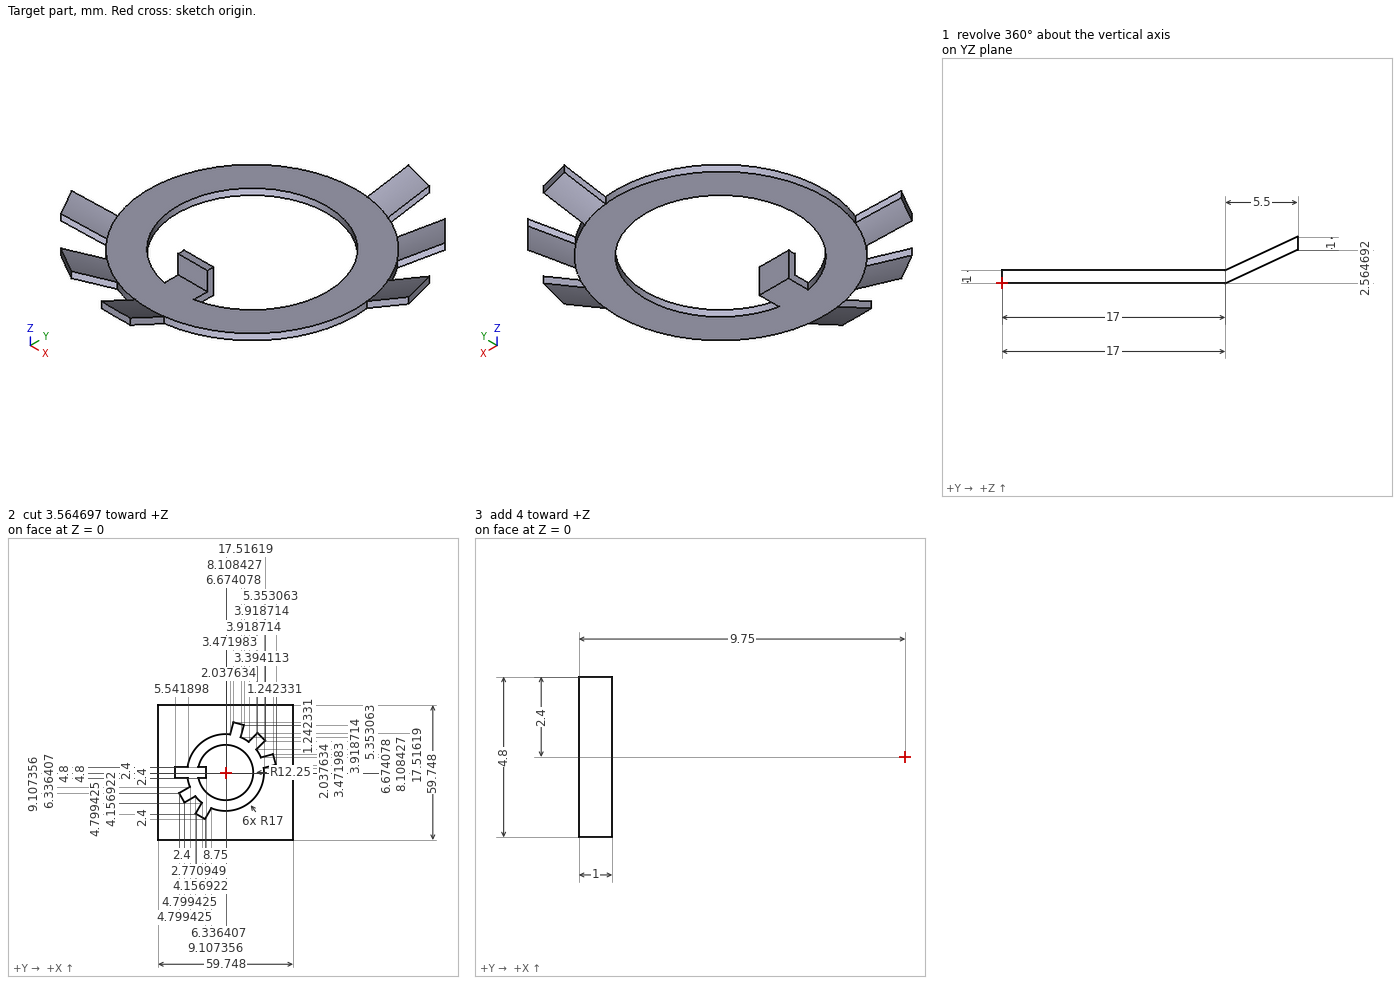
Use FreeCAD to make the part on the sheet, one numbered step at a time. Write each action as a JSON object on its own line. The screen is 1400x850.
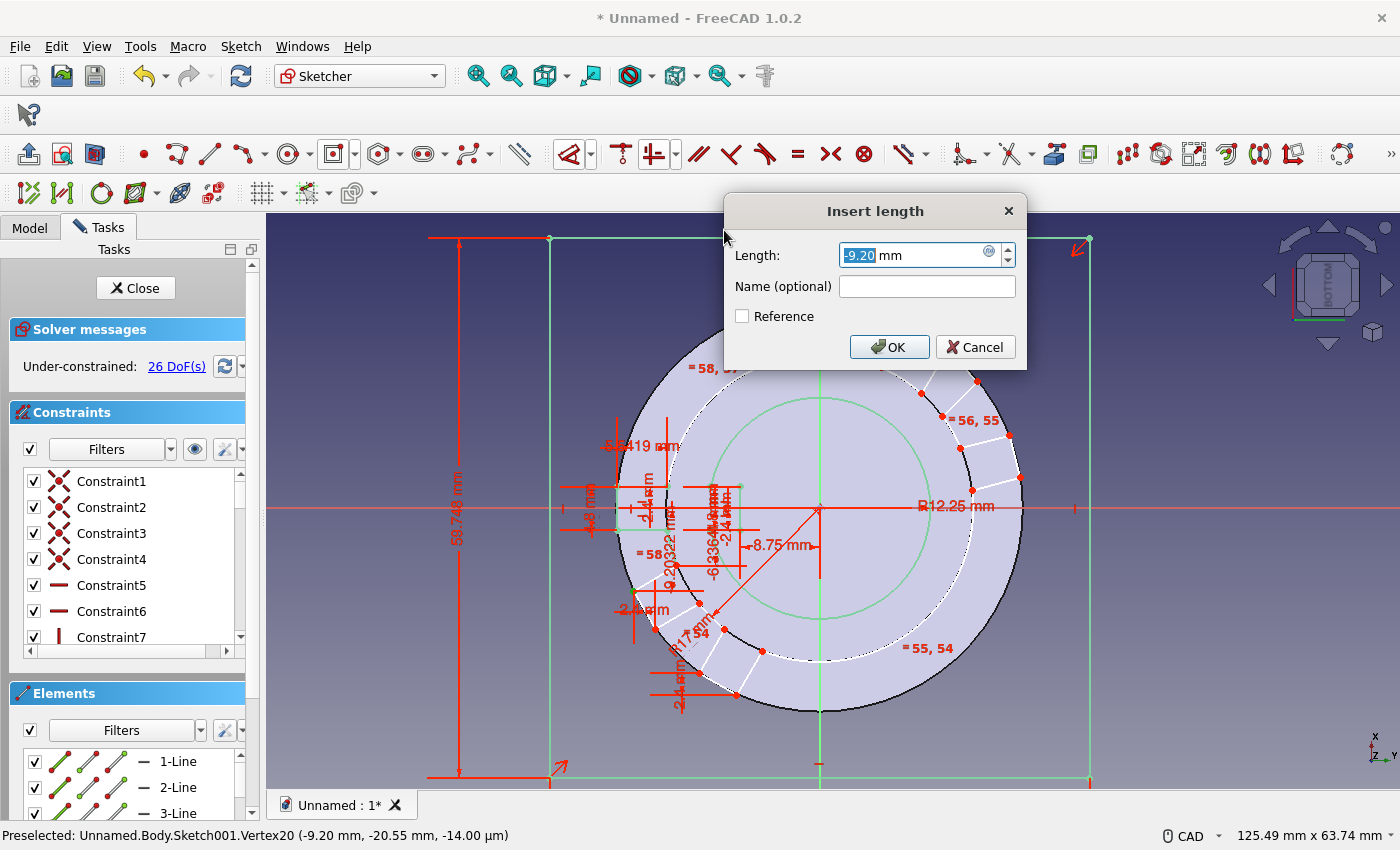
{"action": "type", "text": "-9.107356"}
{"action": "key", "text": "Return"}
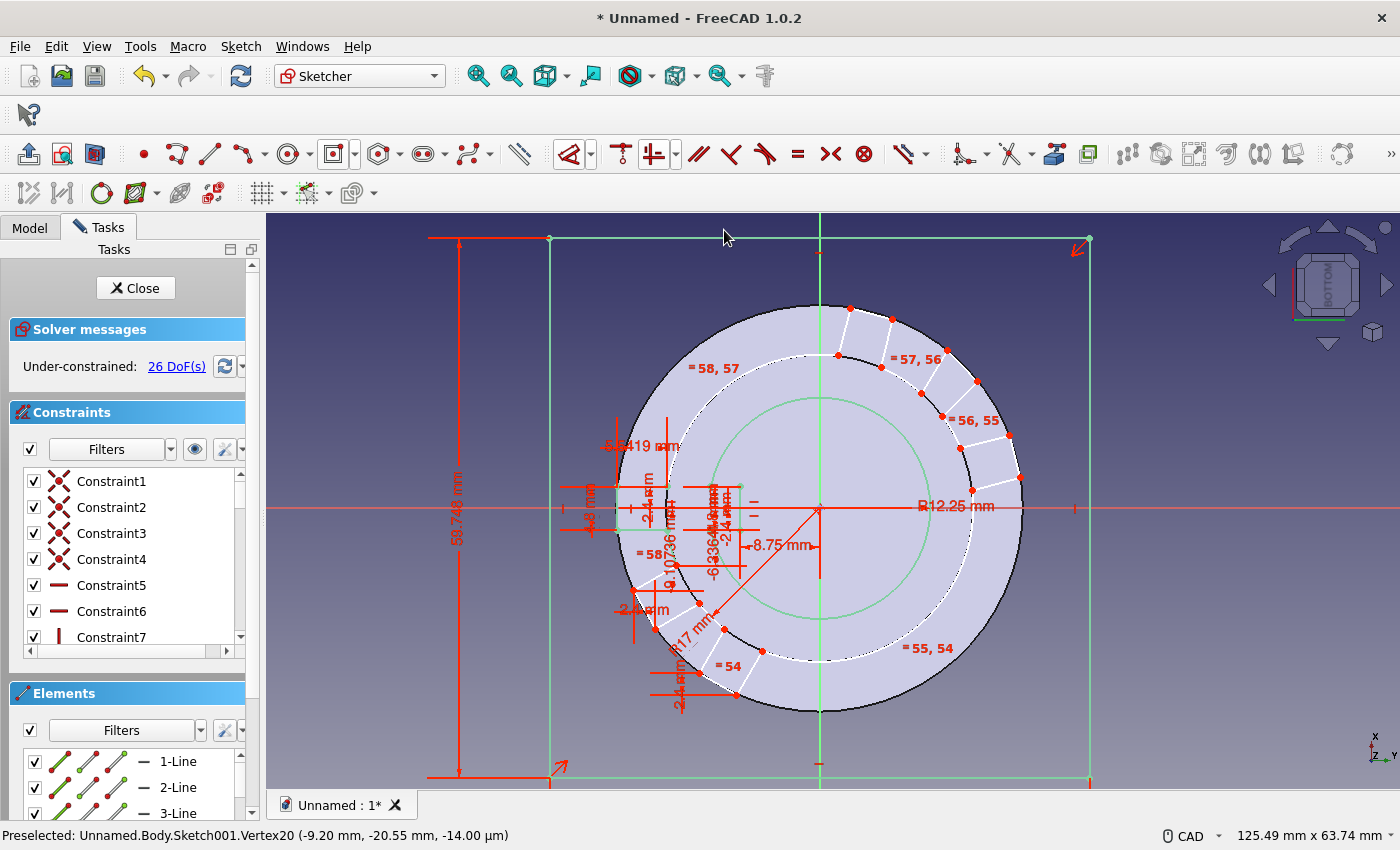
{"action": "left_click", "coordinate": [737, 695]}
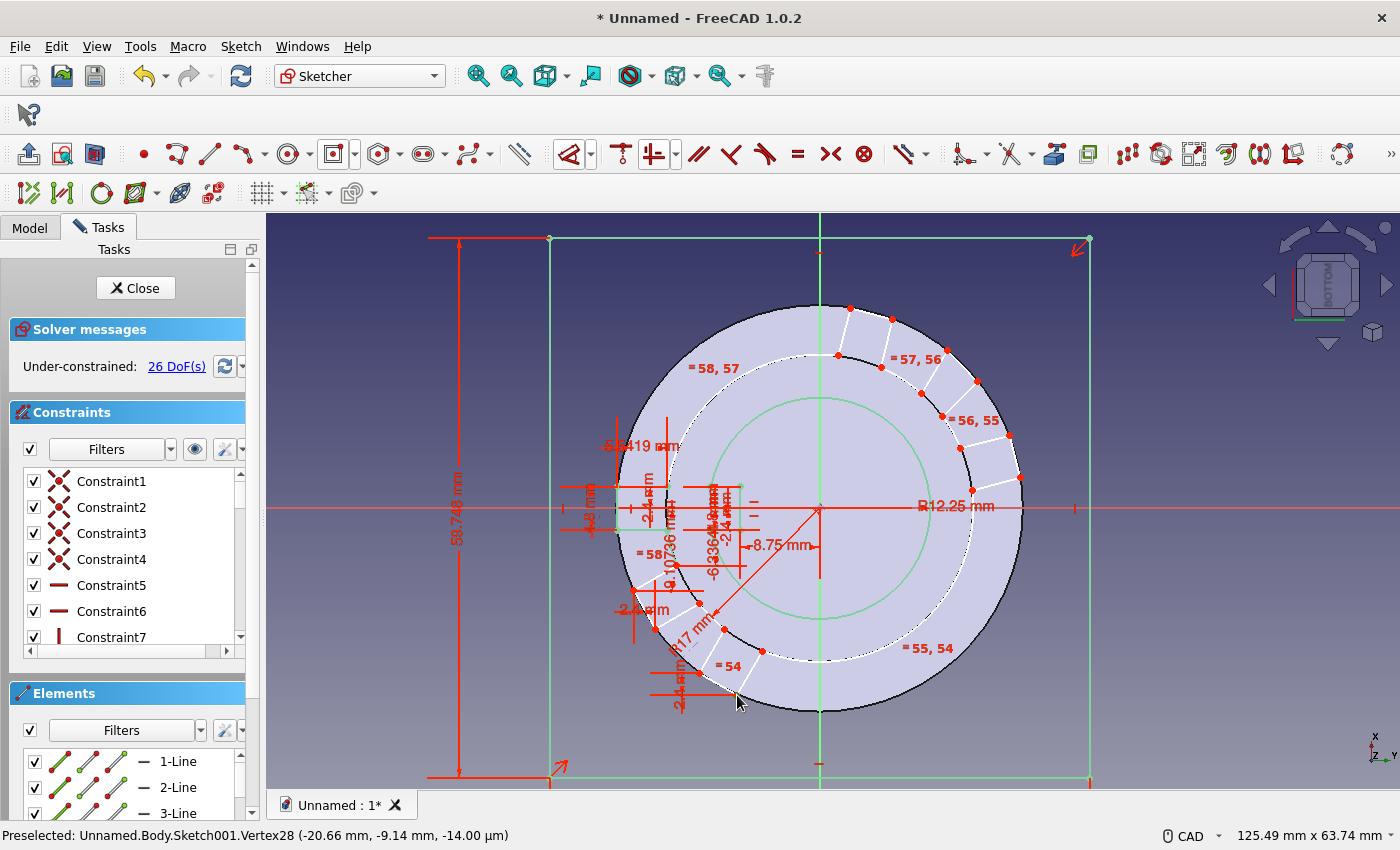
{"action": "left_click", "coordinate": [590, 154]}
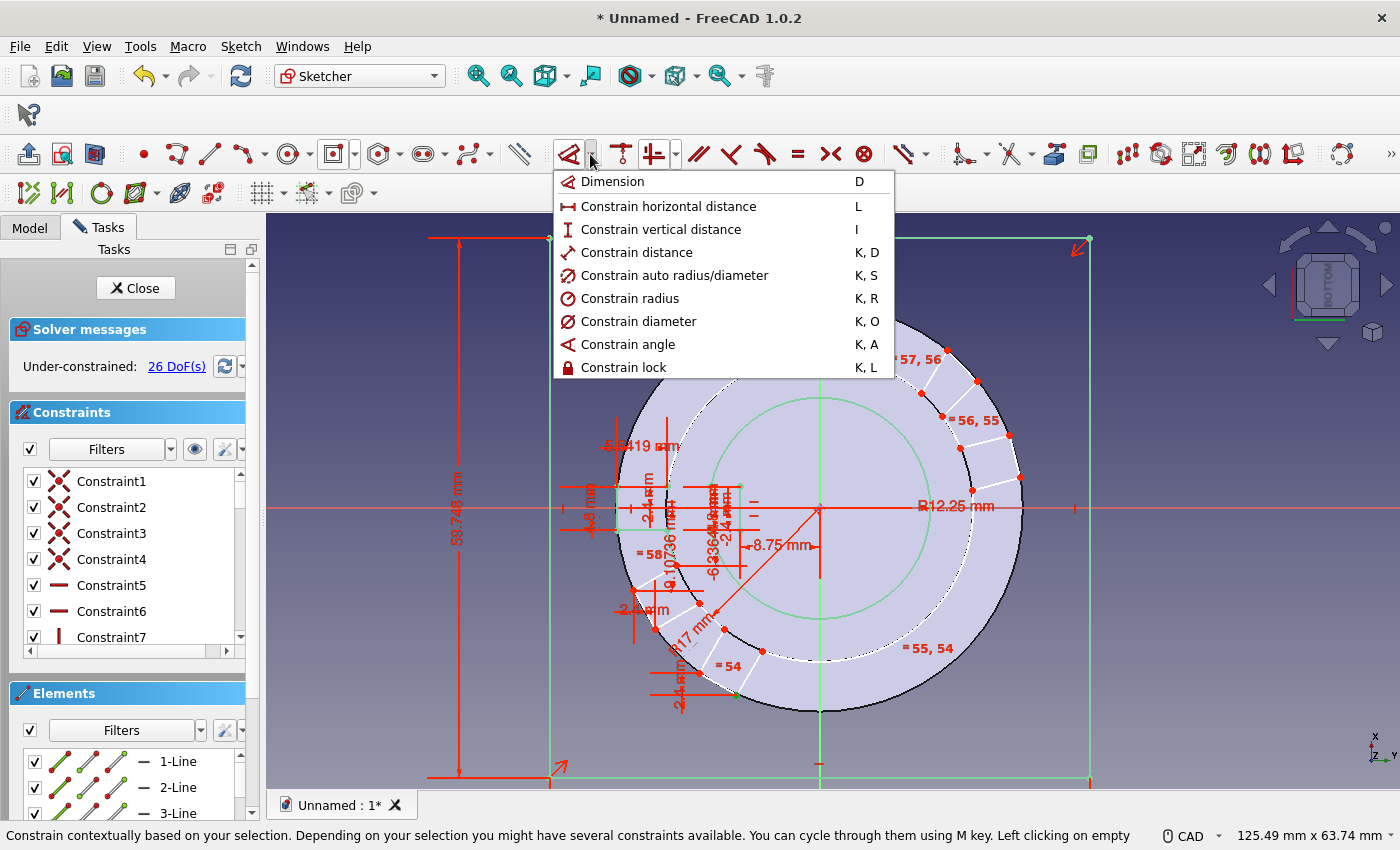
{"action": "left_click", "coordinate": [724, 206]}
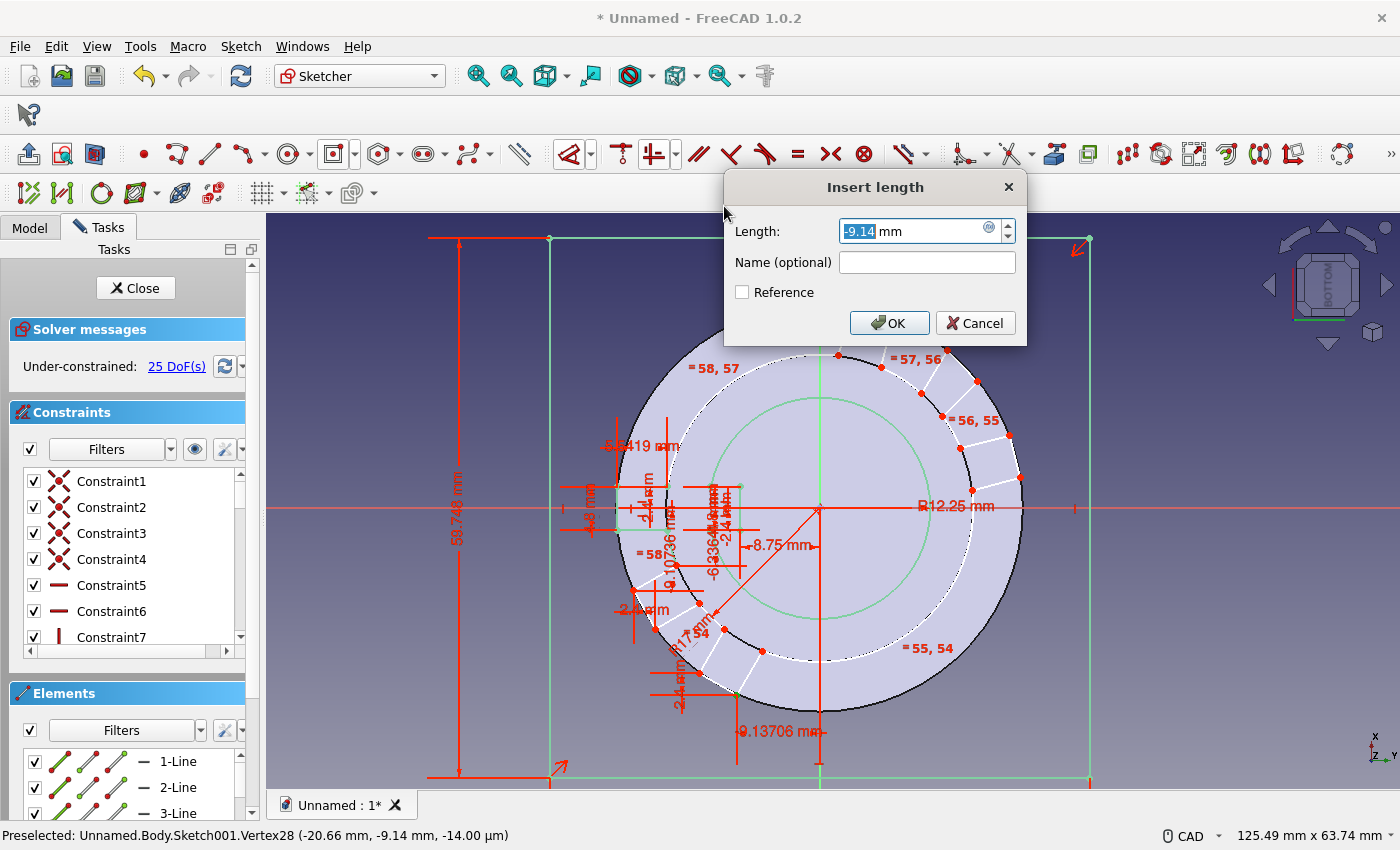
{"action": "type", "text": "-9.107356"}
{"action": "key", "text": "Return"}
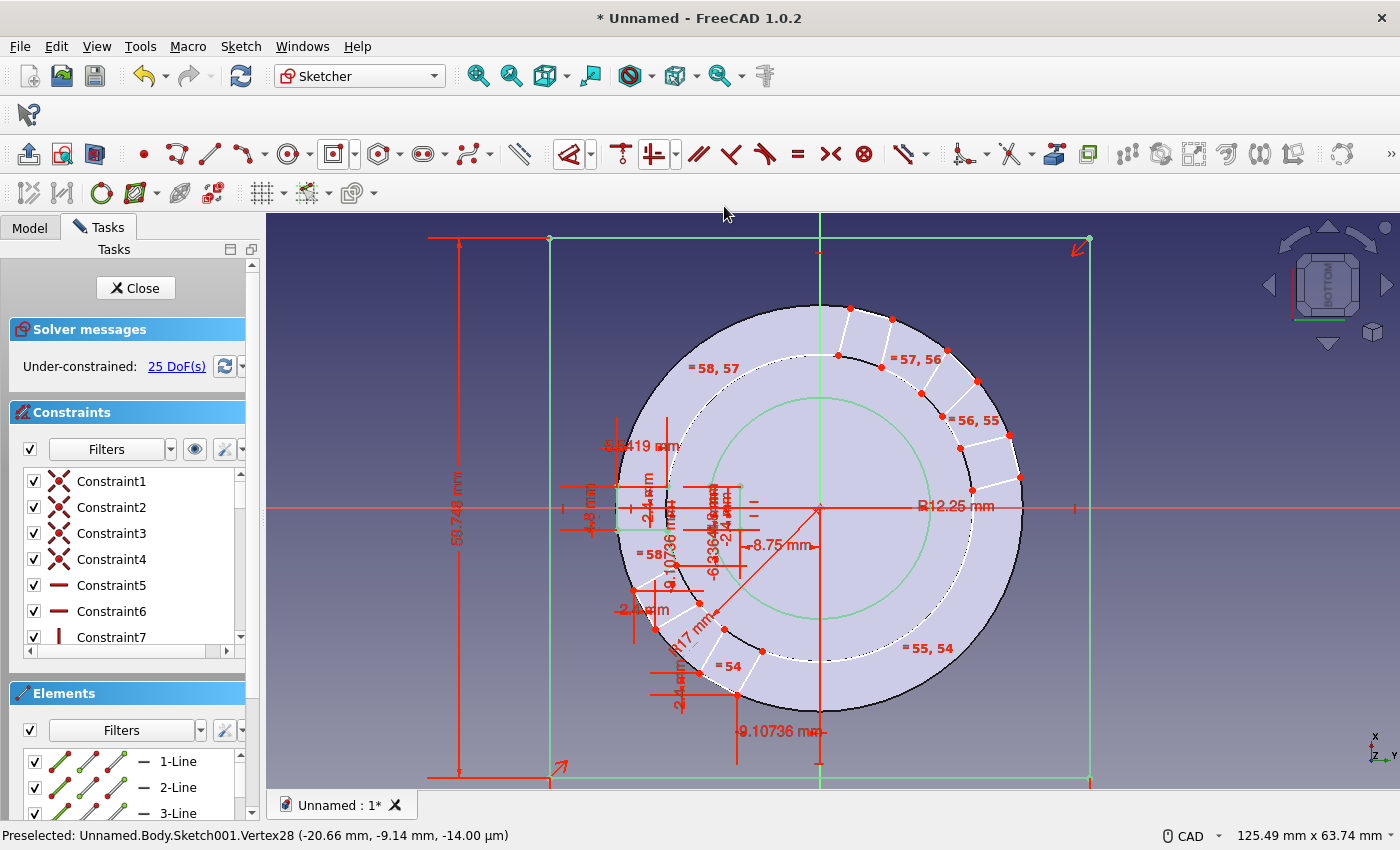
{"action": "left_click", "coordinate": [763, 651]}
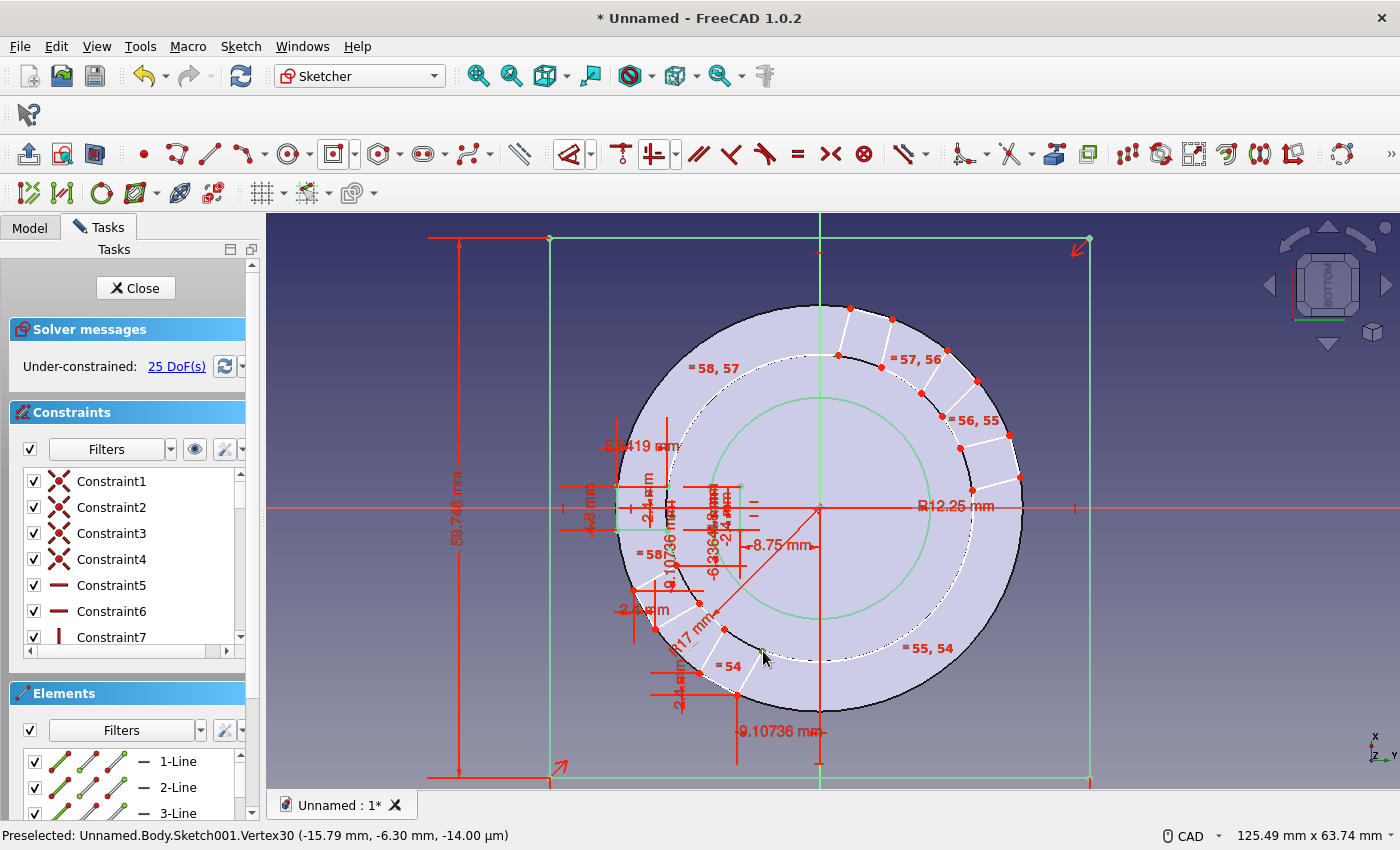
{"action": "key", "text": "l"}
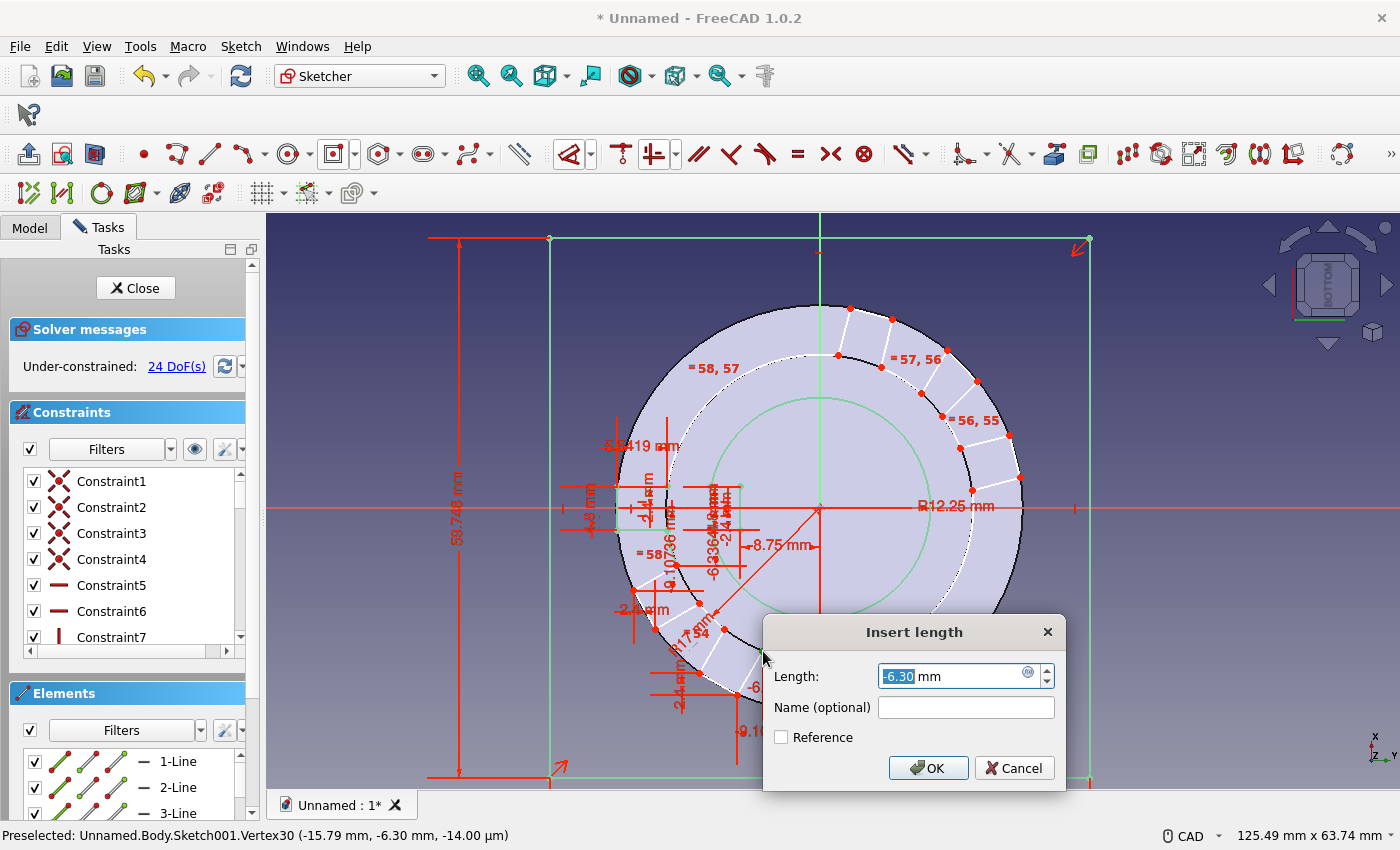
{"action": "type", "text": "-6.336407"}
{"action": "key", "text": "Return"}